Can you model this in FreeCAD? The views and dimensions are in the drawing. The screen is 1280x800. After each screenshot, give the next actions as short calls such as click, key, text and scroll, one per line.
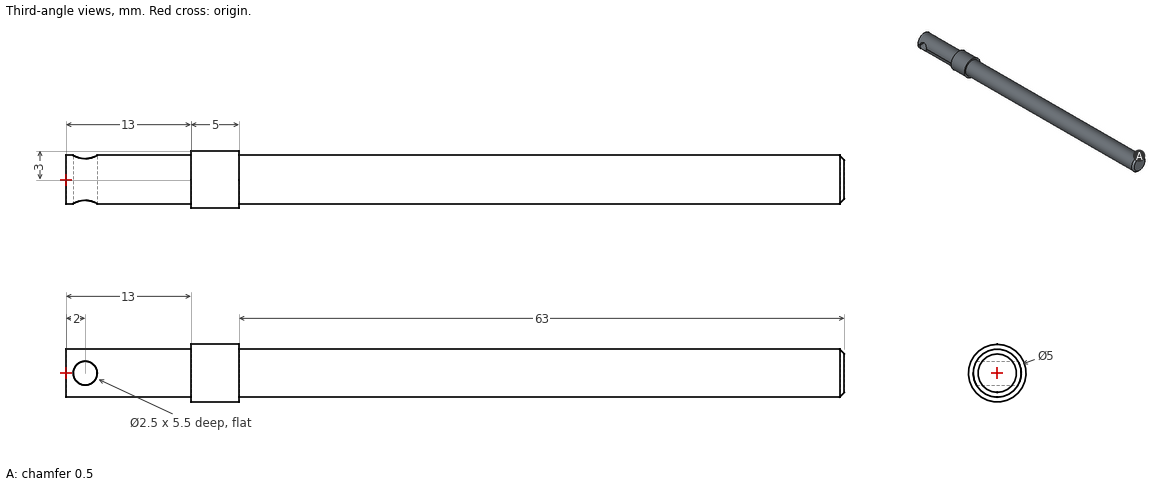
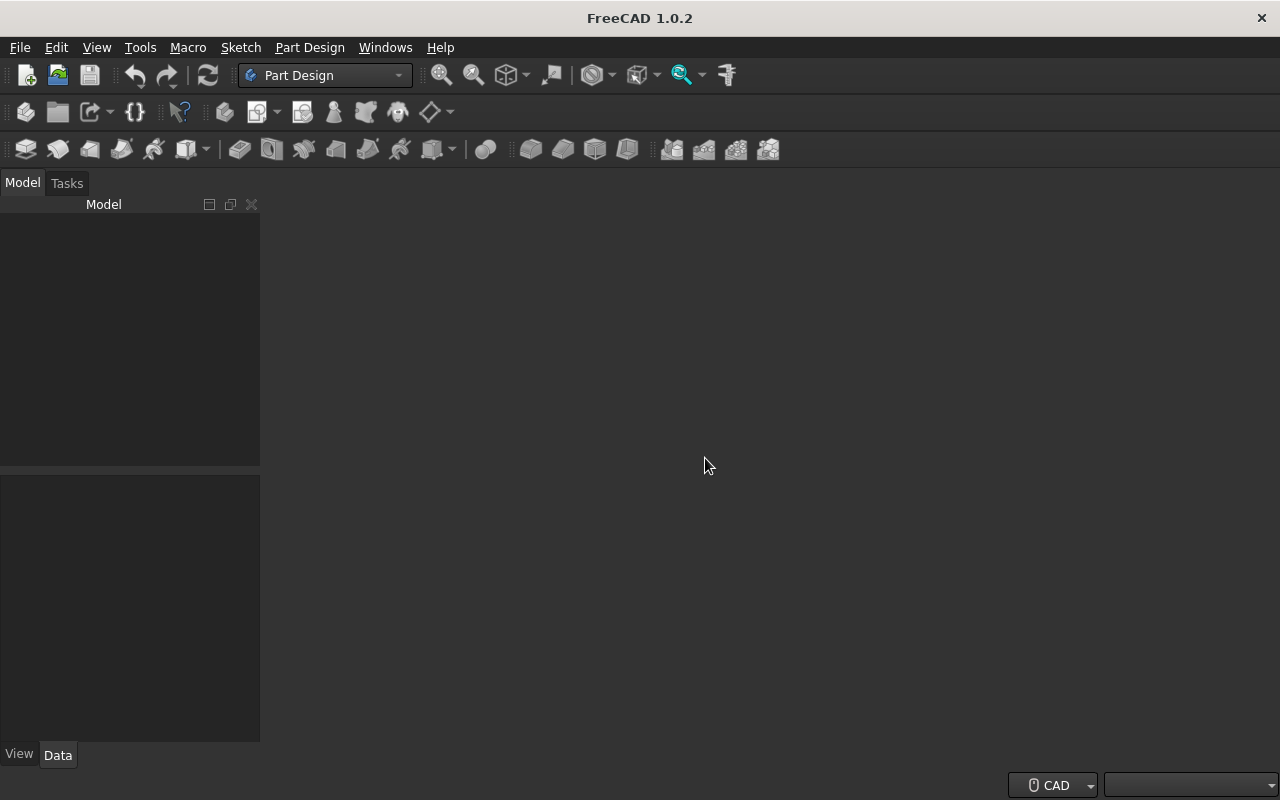
click(26, 76)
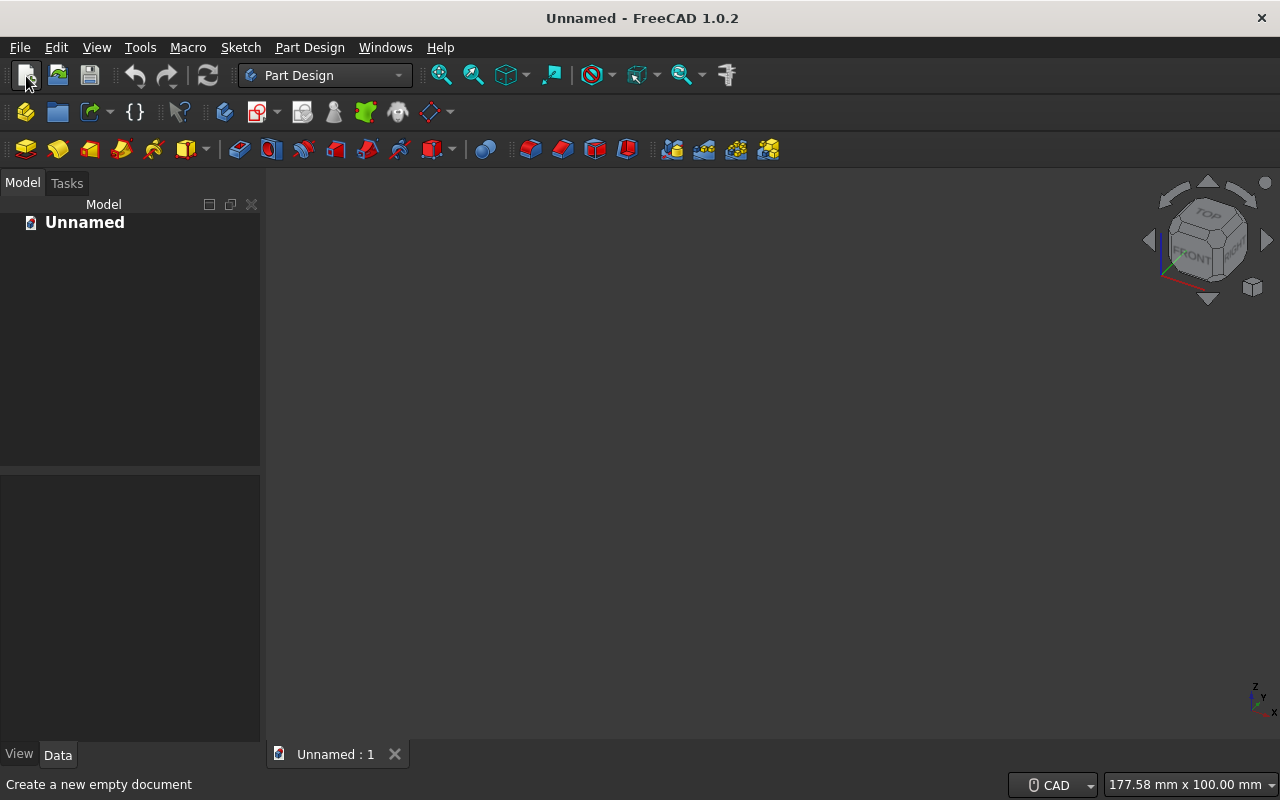
click(258, 112)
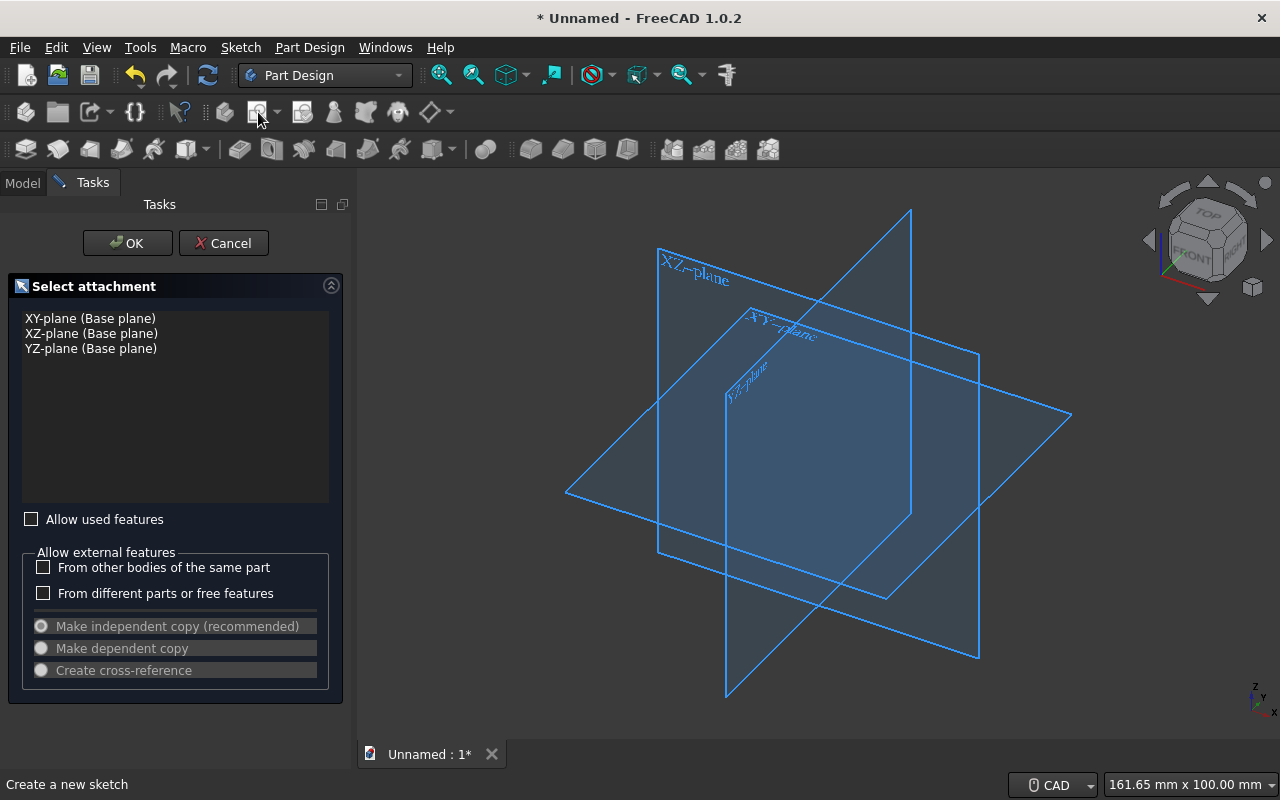
click(82, 318)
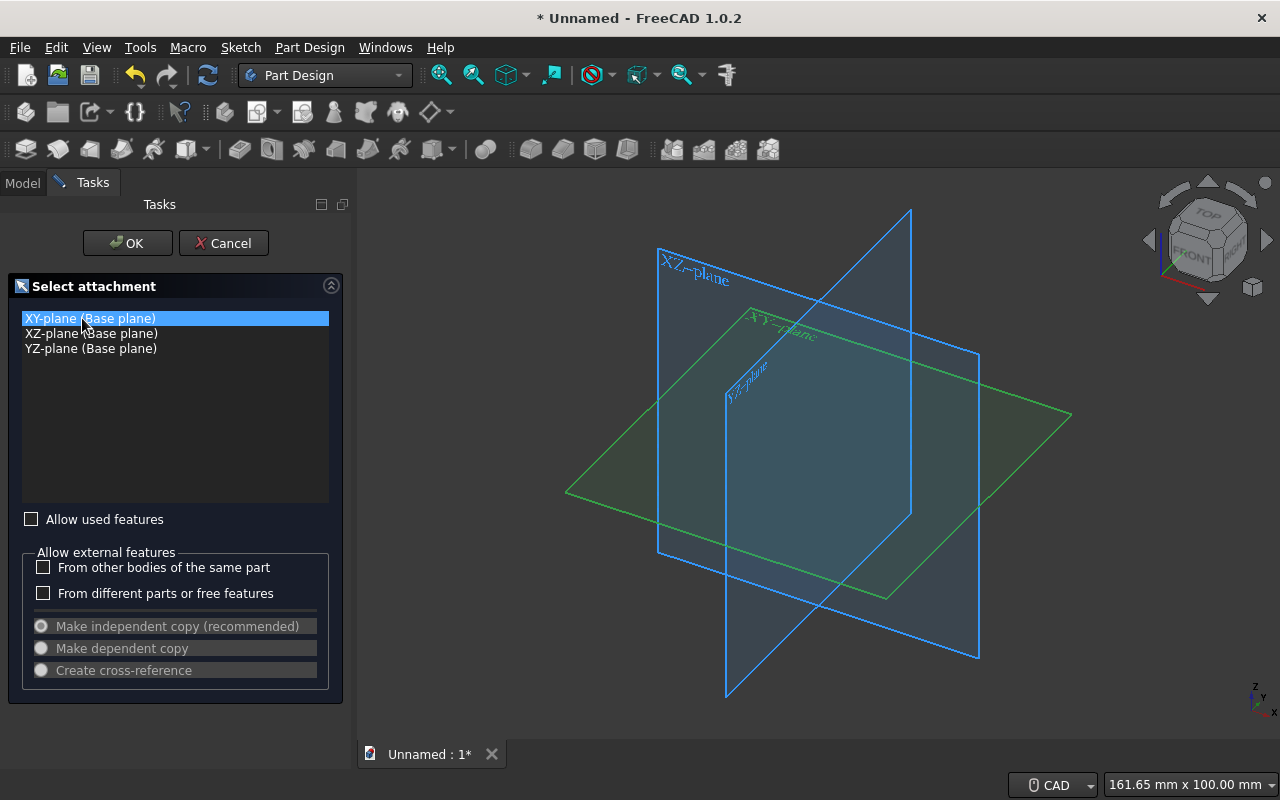
click(128, 243)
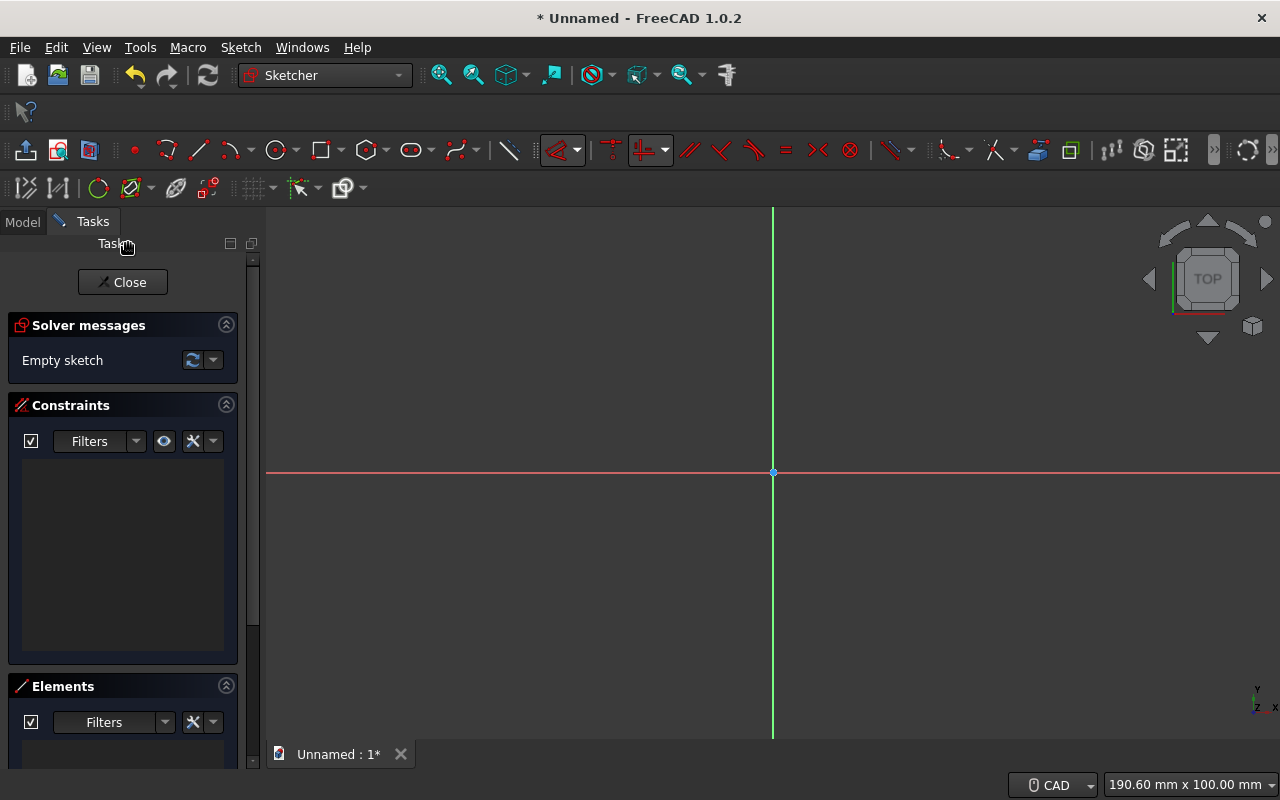
scroll(863, 465, up, 15)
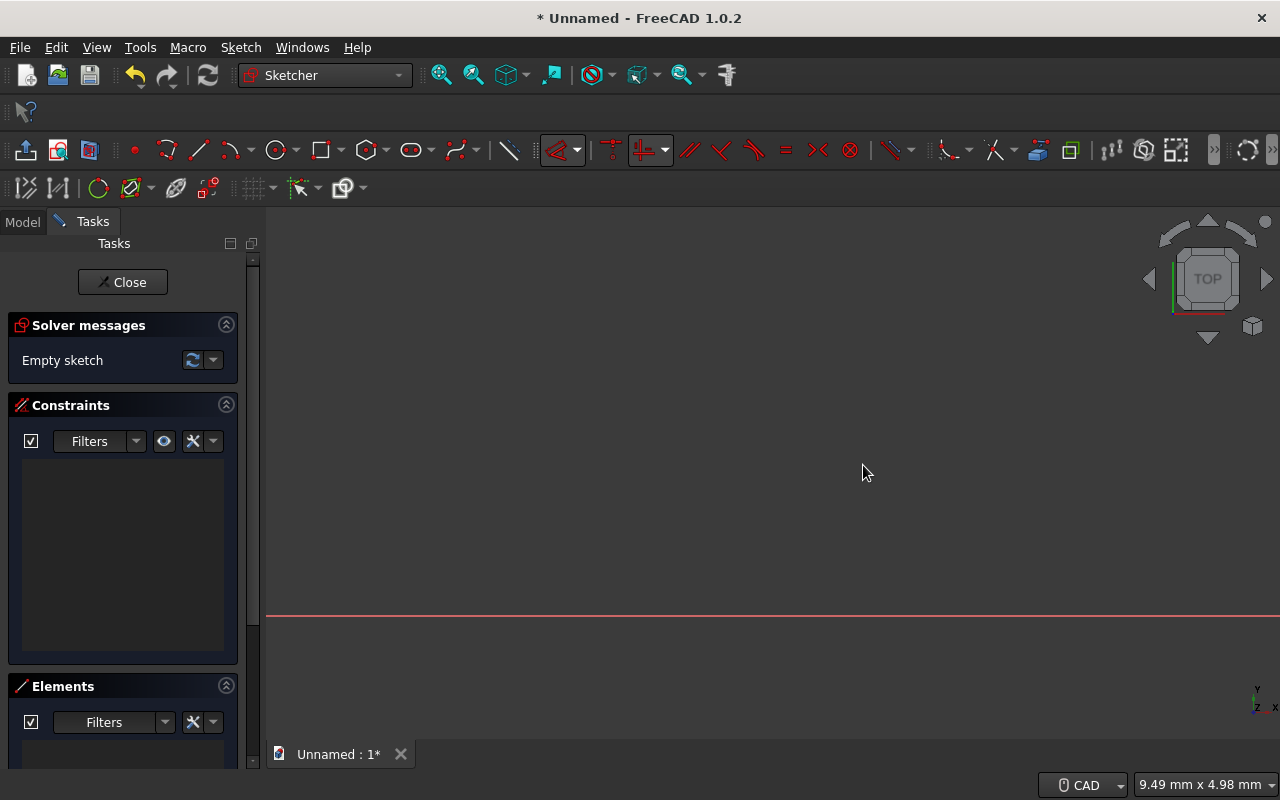
click(322, 150)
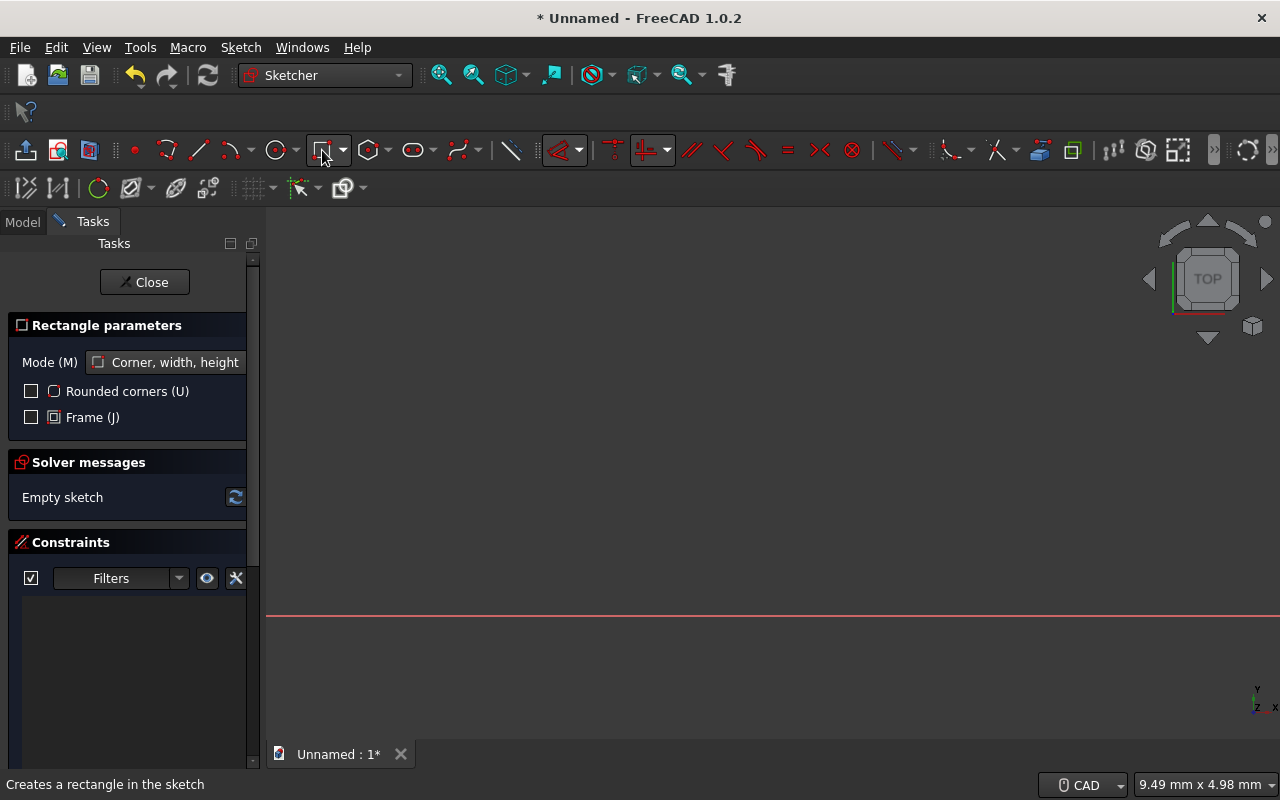
click(433, 296)
click(967, 616)
key(Escape)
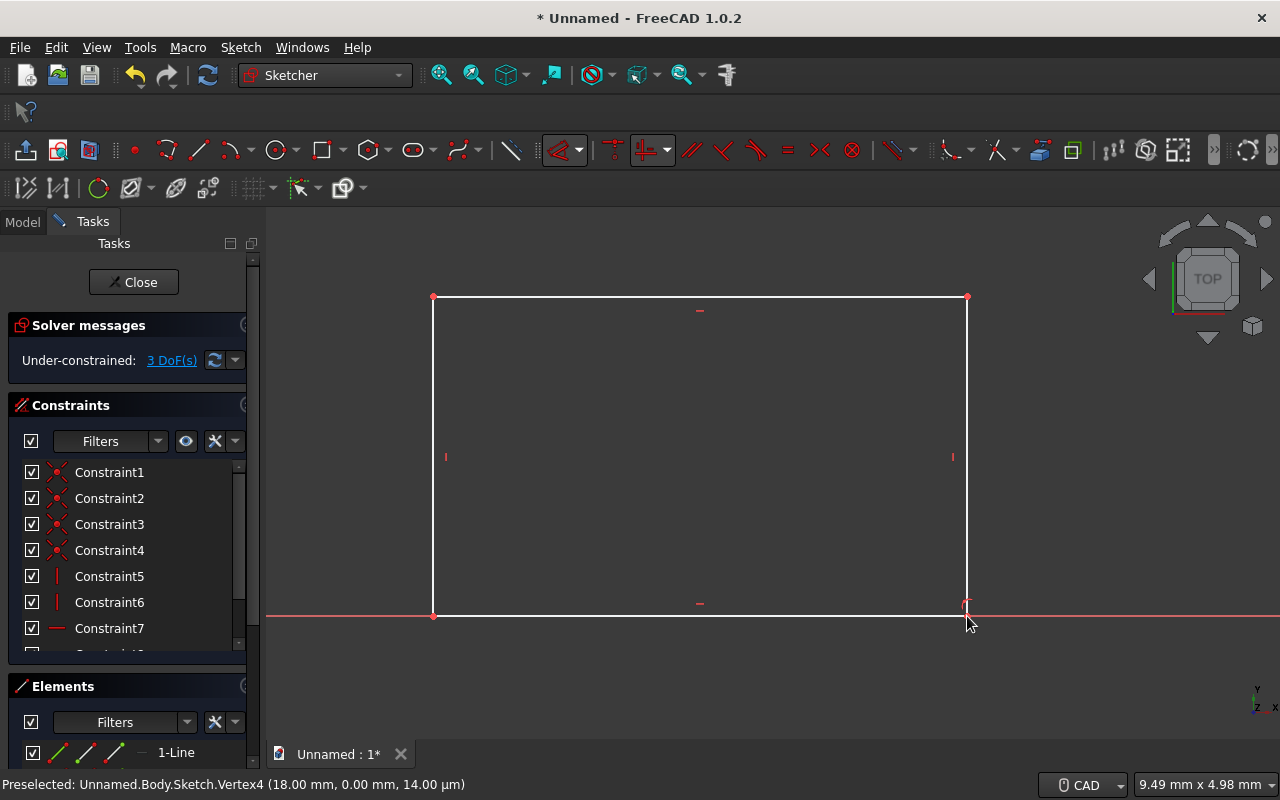
click(558, 150)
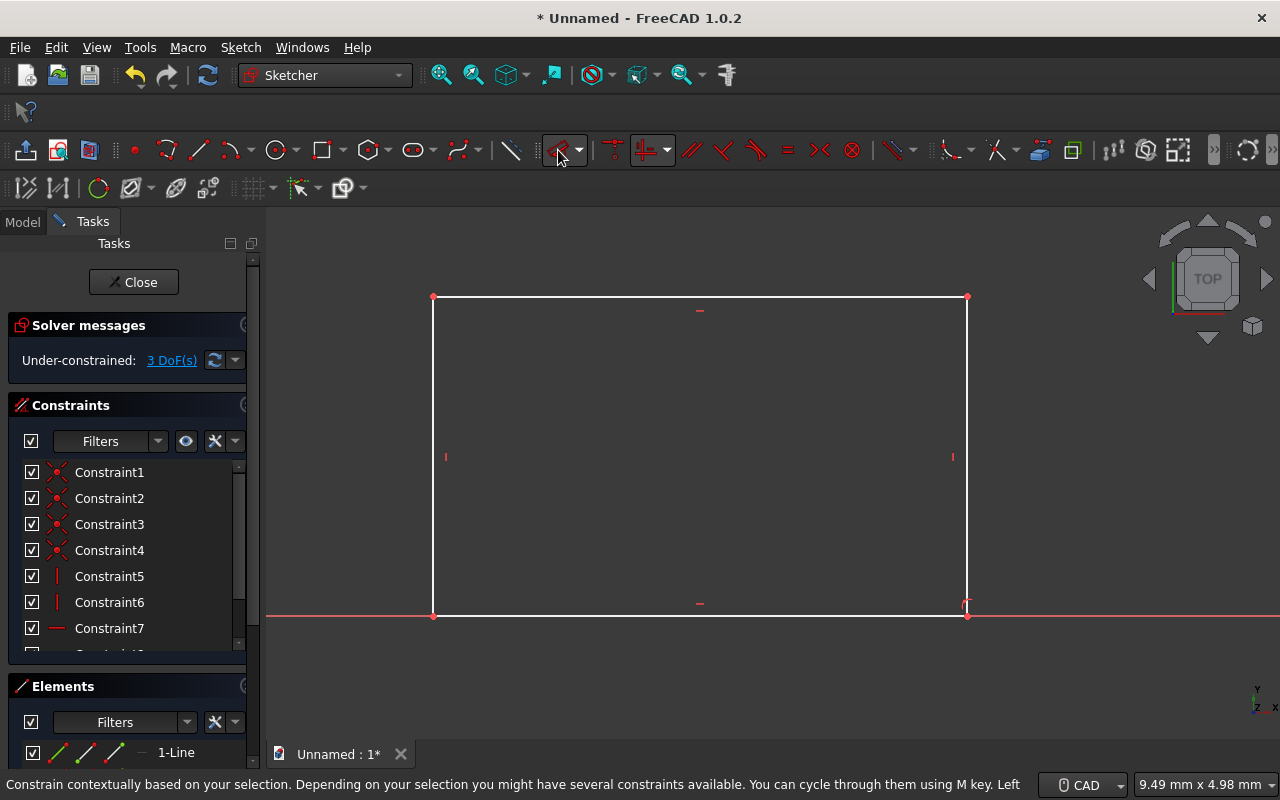
click(433, 393)
click(399, 457)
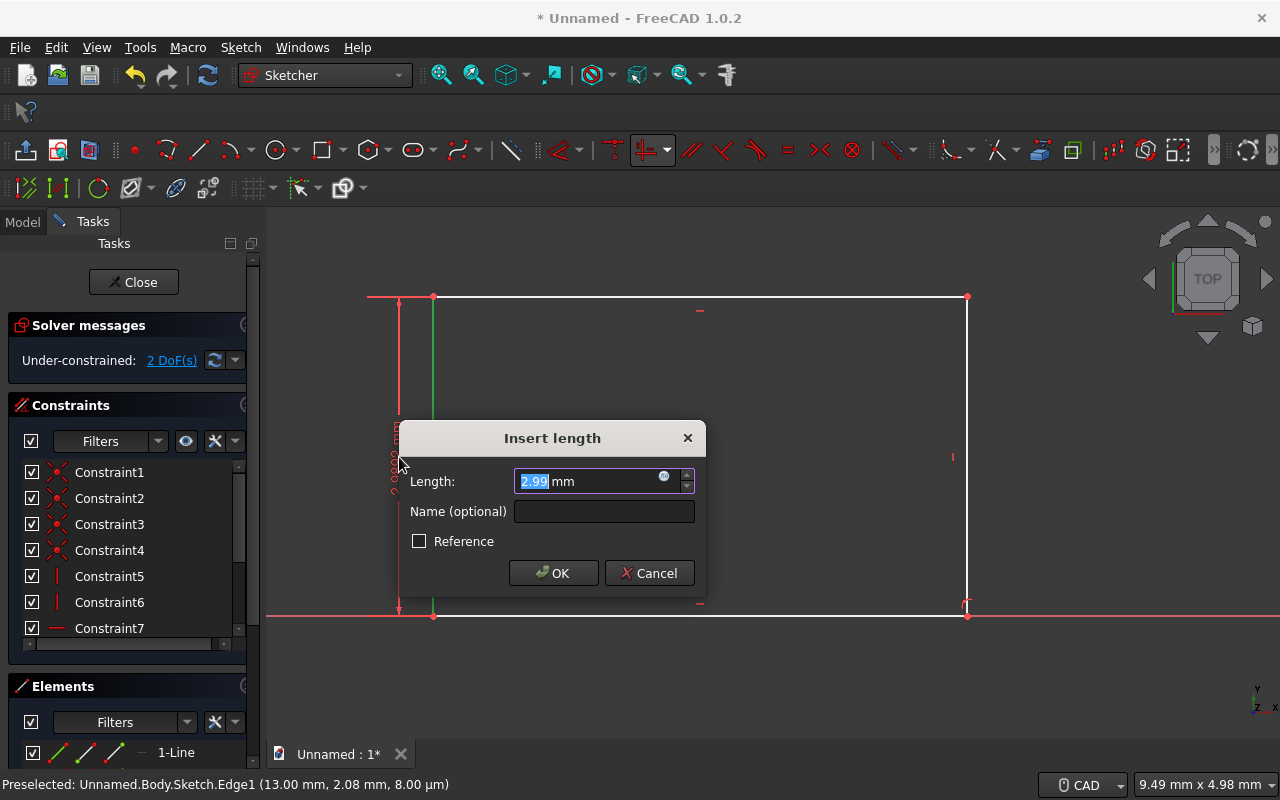
text(3)
key(Return)